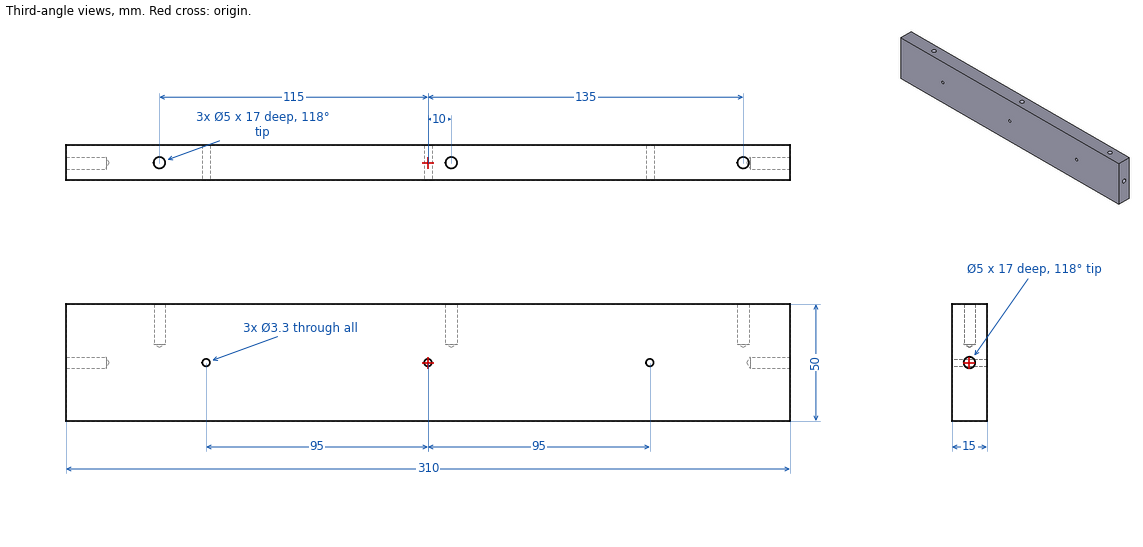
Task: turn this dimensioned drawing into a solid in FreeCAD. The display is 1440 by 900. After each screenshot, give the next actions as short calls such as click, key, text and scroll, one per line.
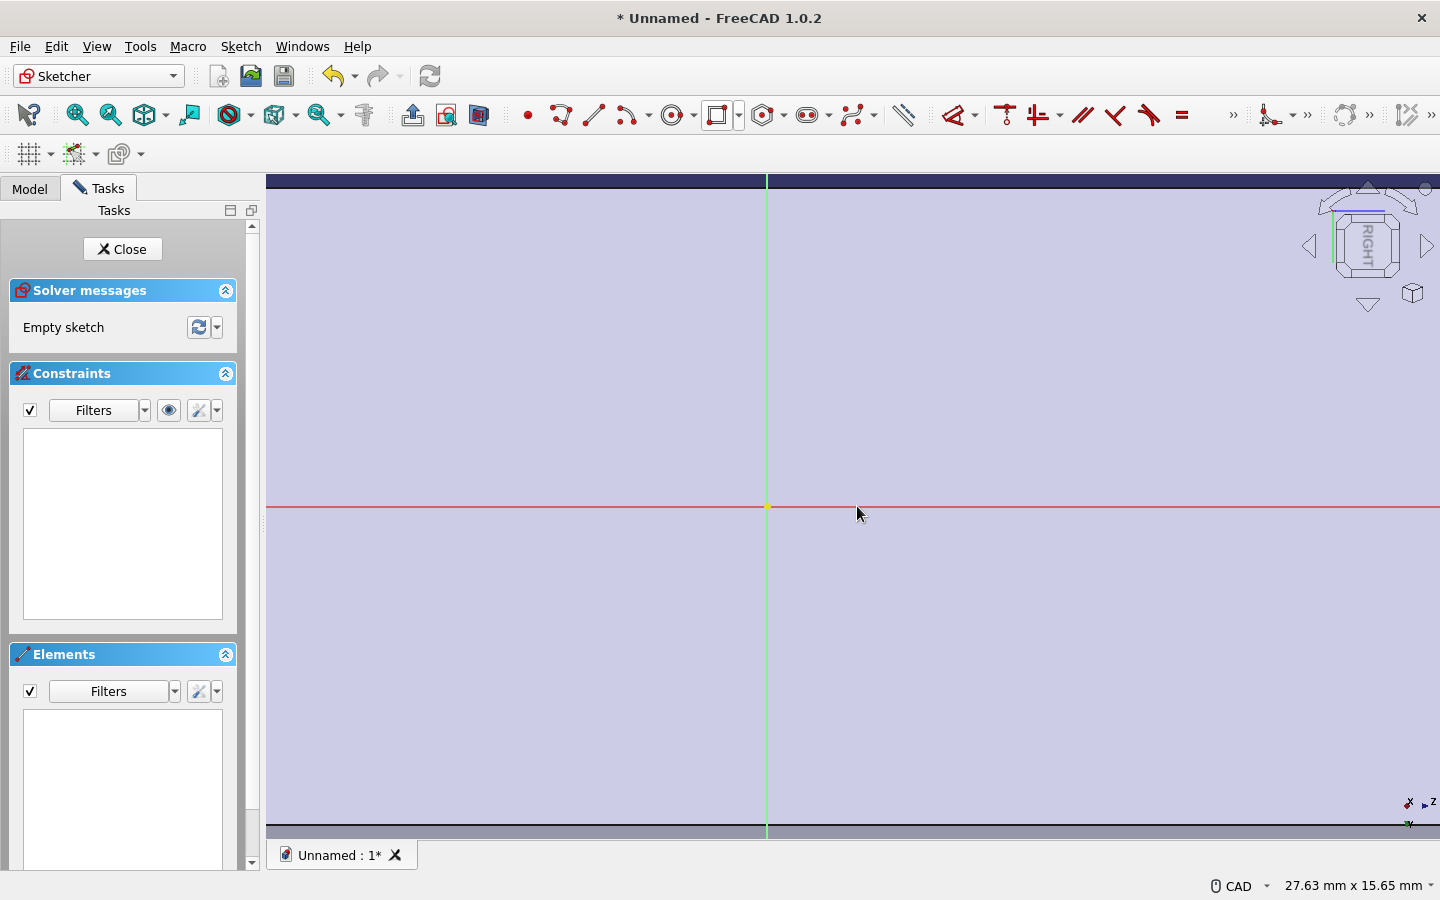
scroll(753, 506, up, 4)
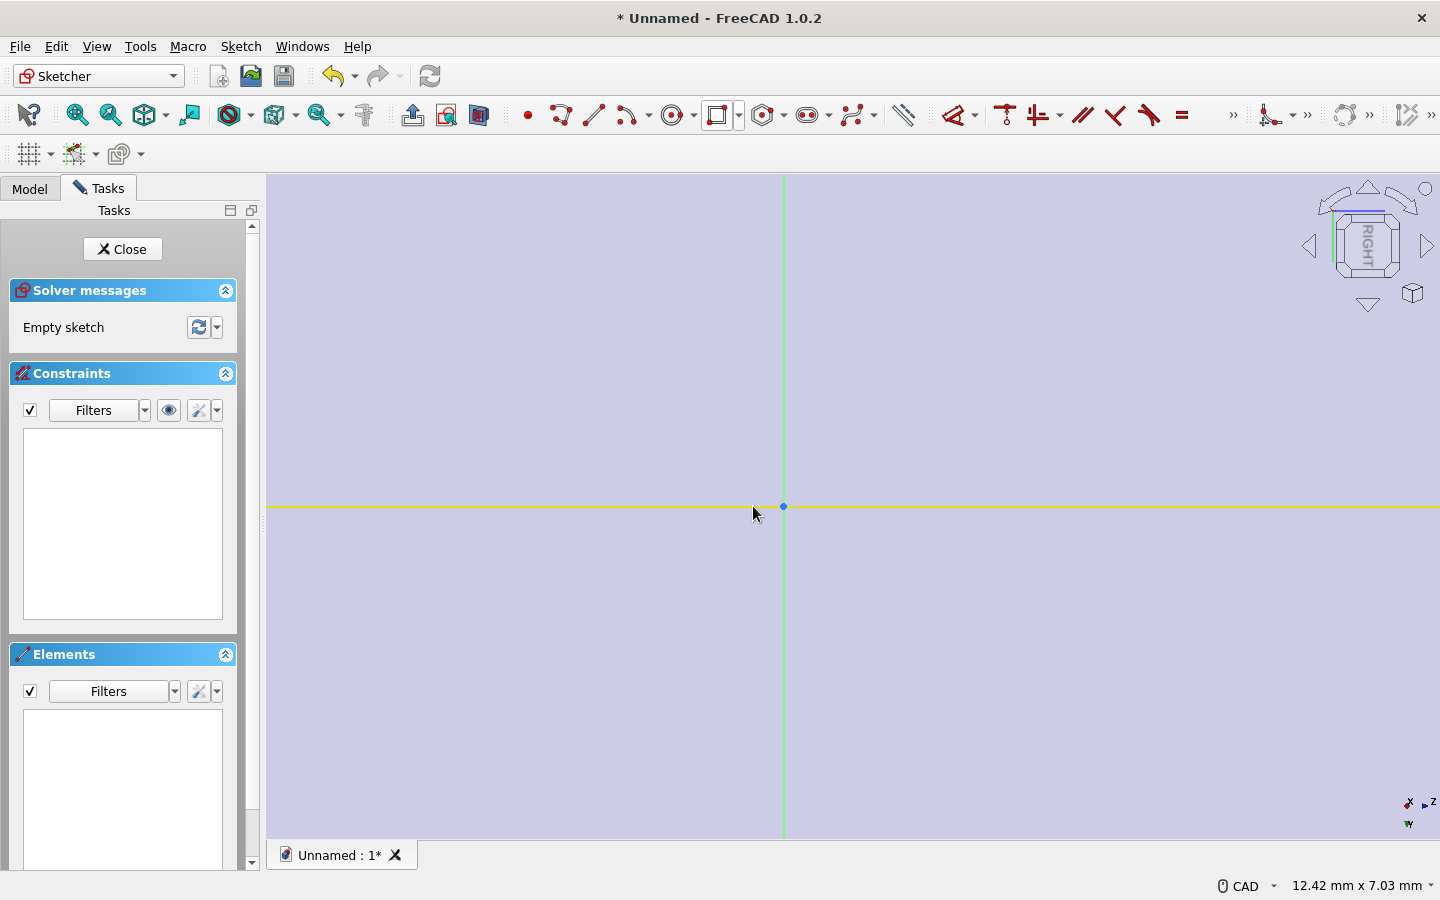
click(672, 116)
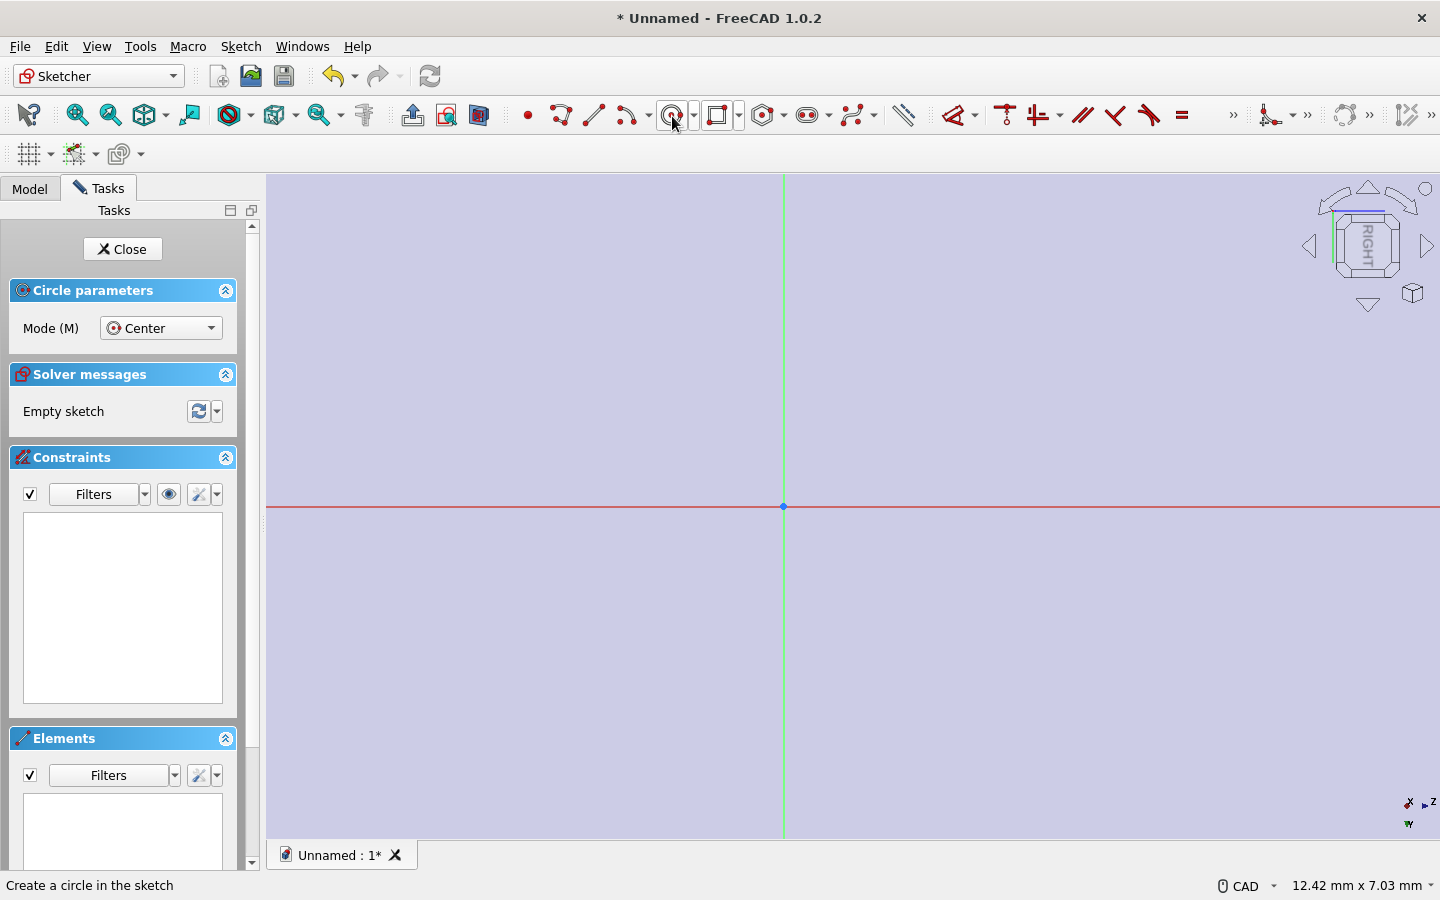
click(784, 506)
click(951, 339)
key(Escape)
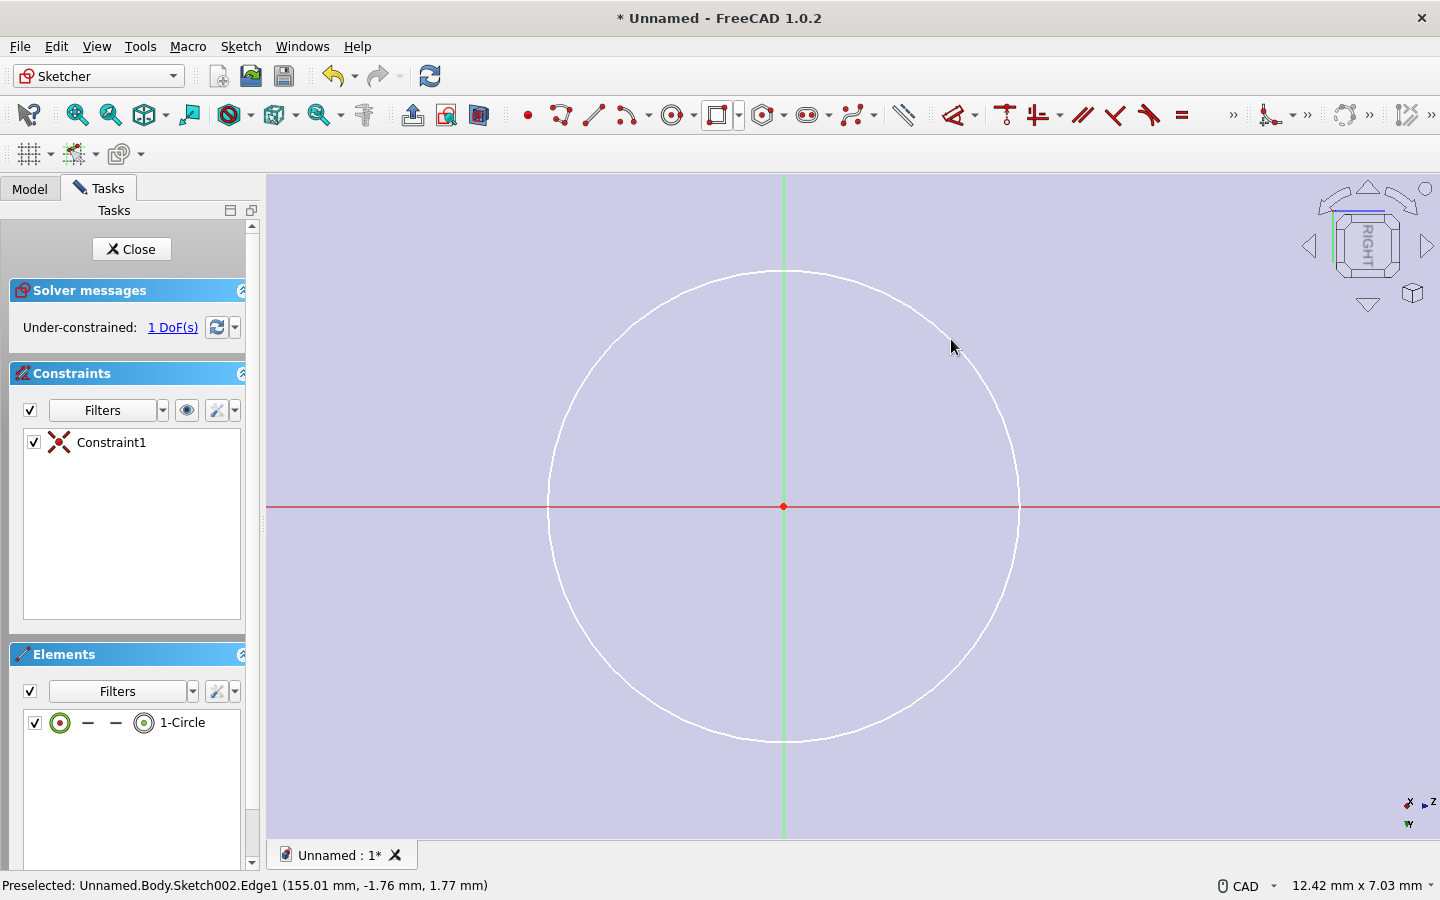
click(952, 116)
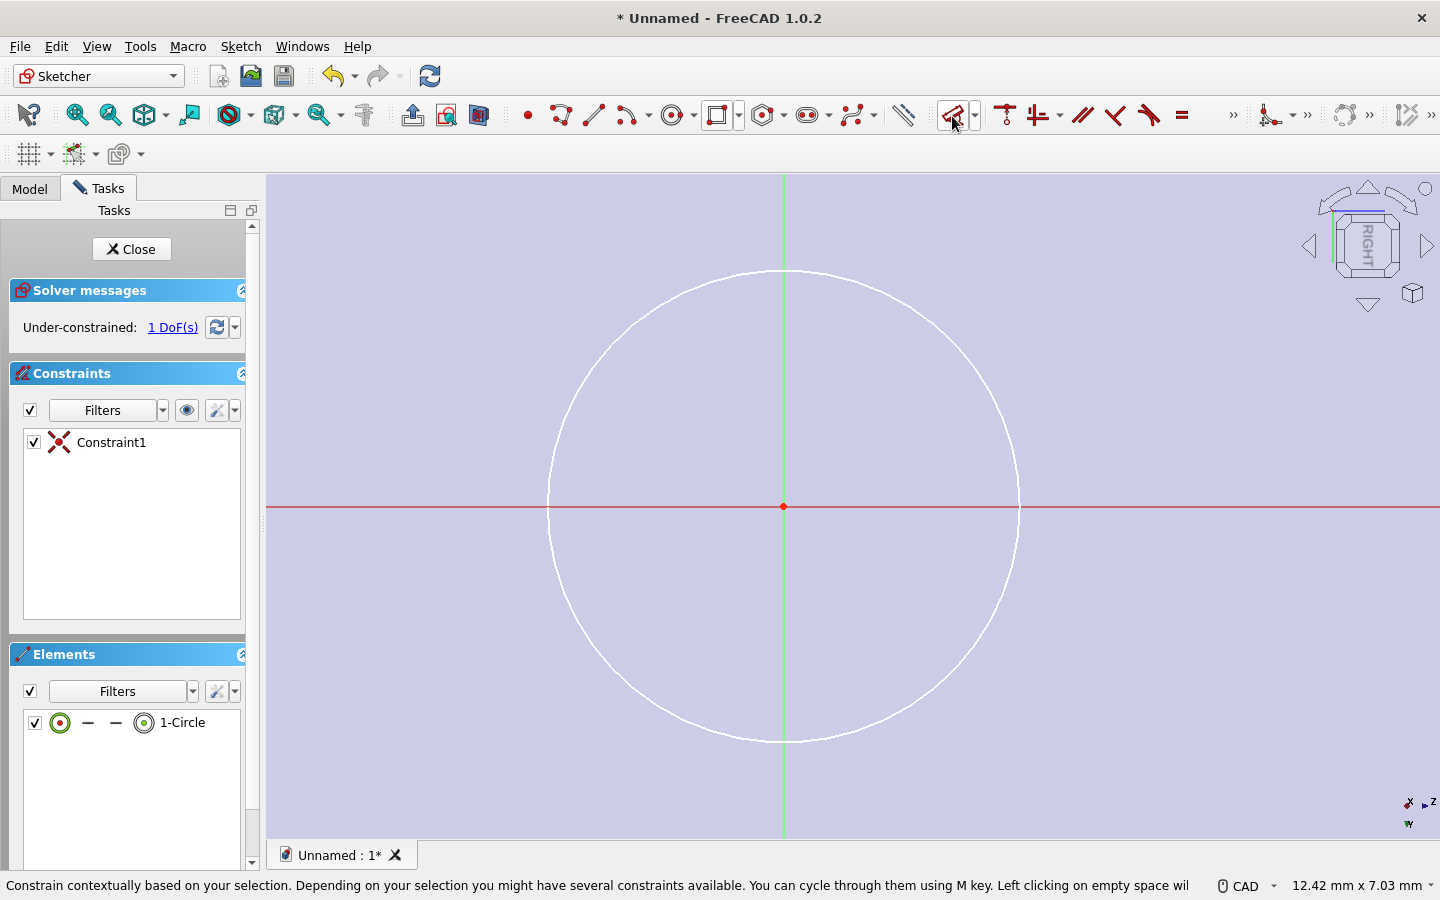
click(950, 339)
click(973, 316)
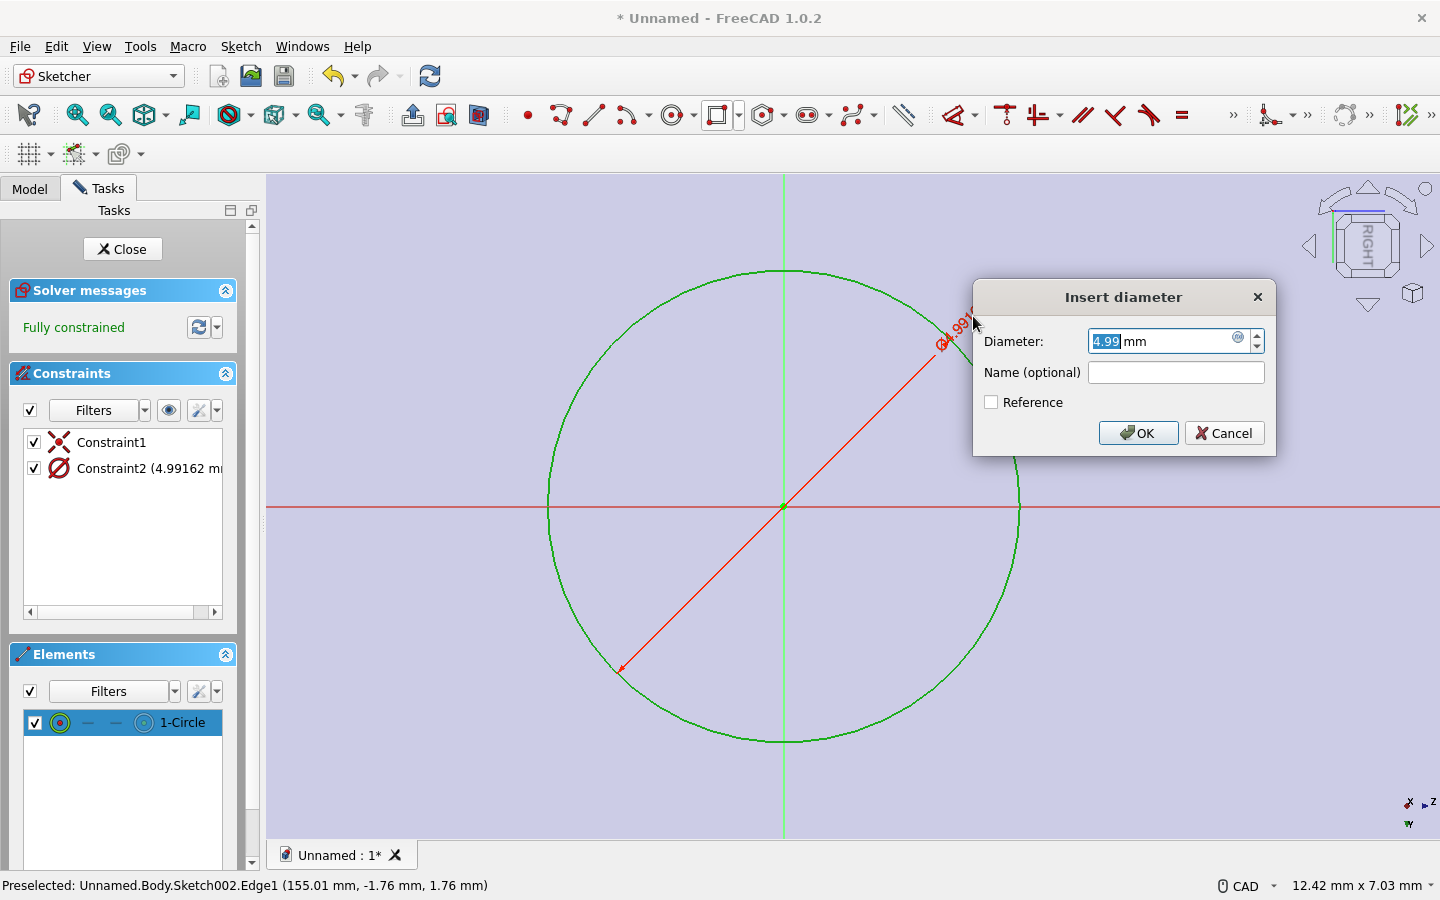
text(5)
key(Return)
key(Escape)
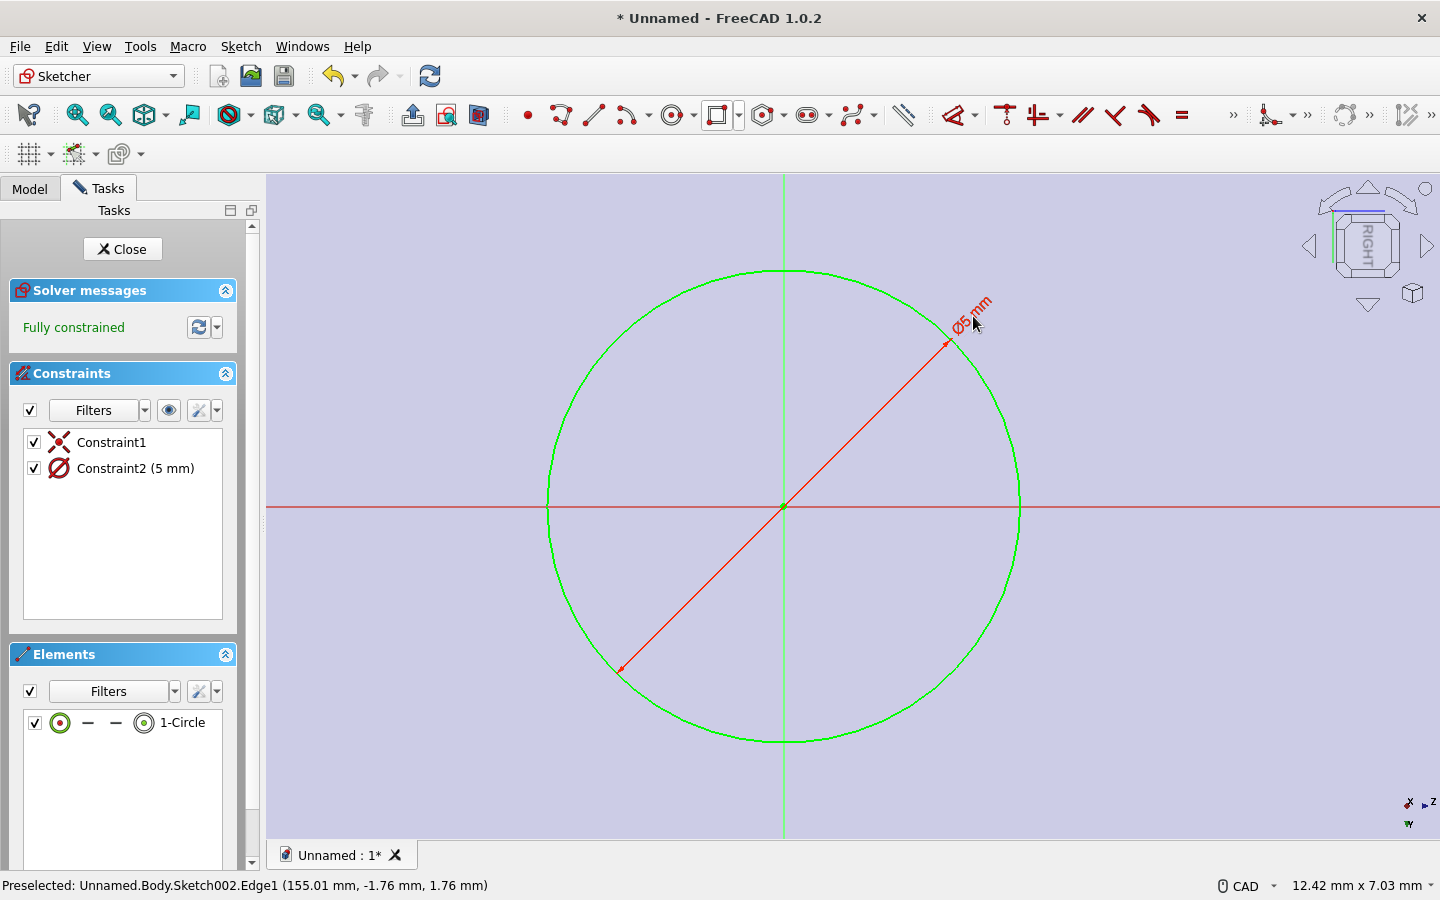
click(123, 249)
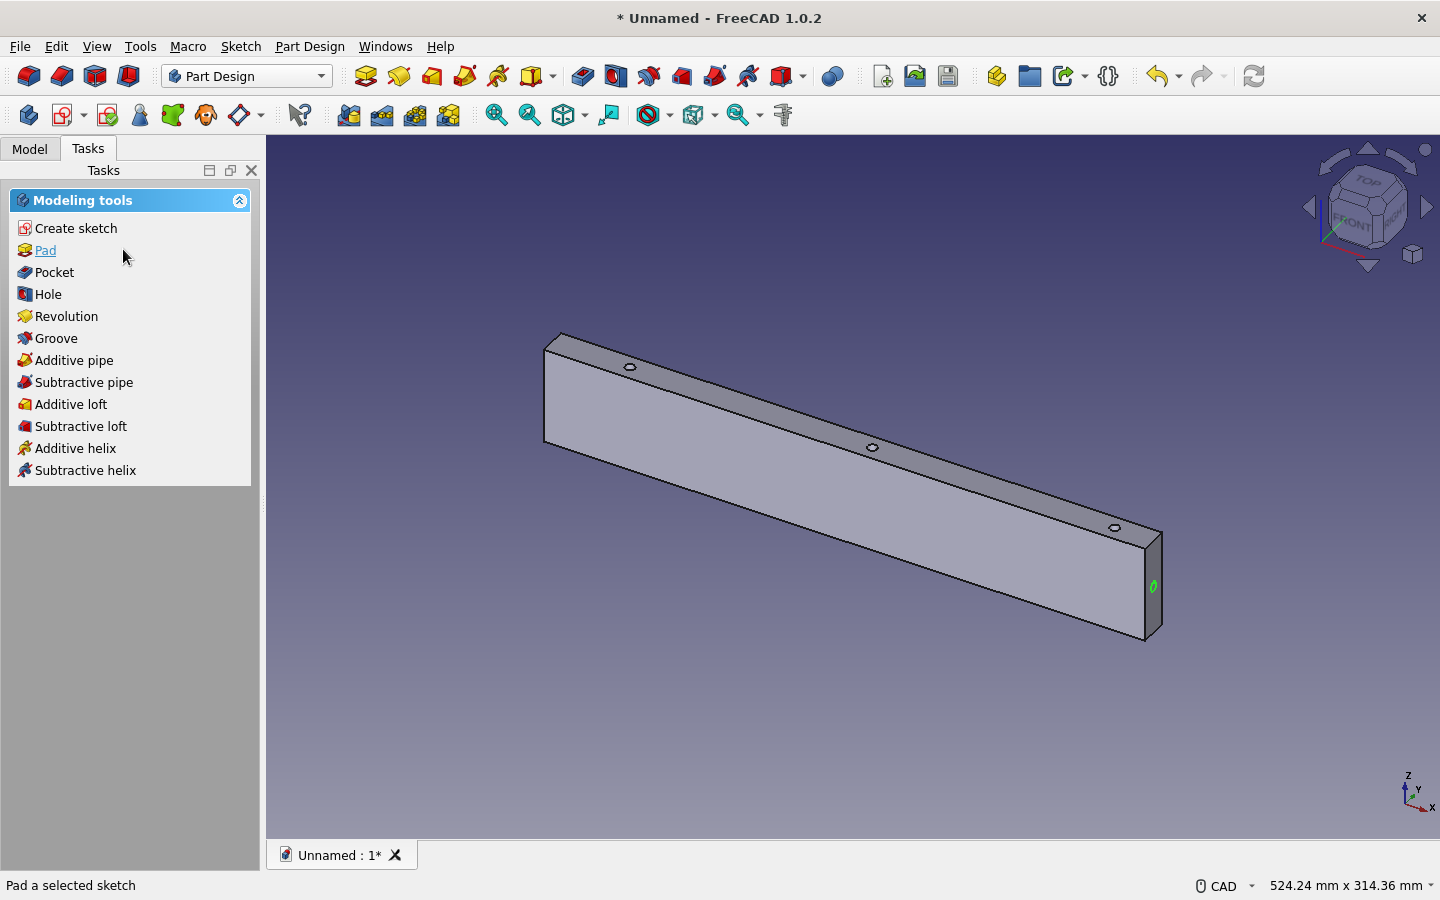
click(616, 76)